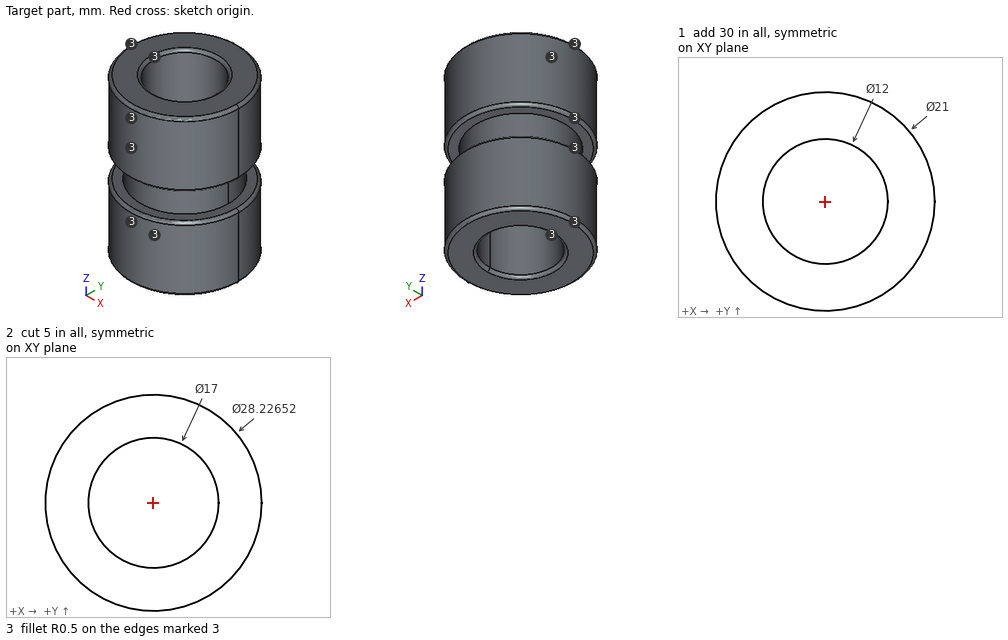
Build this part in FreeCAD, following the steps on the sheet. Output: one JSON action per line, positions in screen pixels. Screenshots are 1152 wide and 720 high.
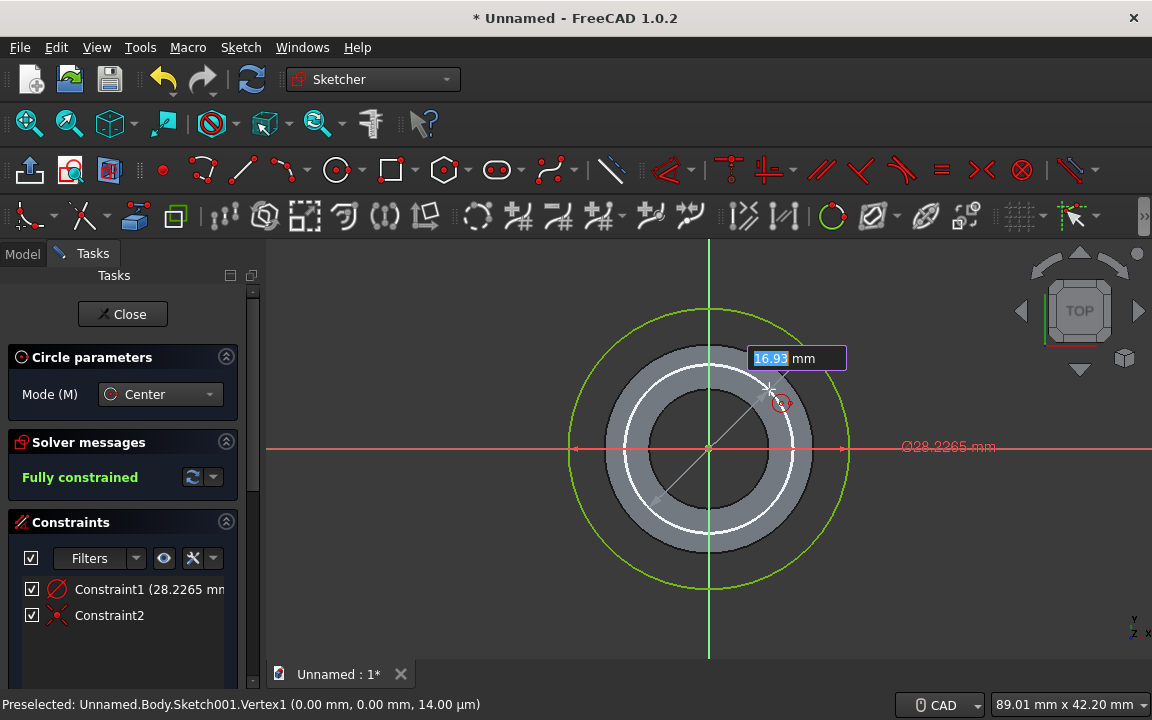
{"action": "type", "text": "17"}
{"action": "key", "text": "Return"}
{"action": "key", "text": "Escape"}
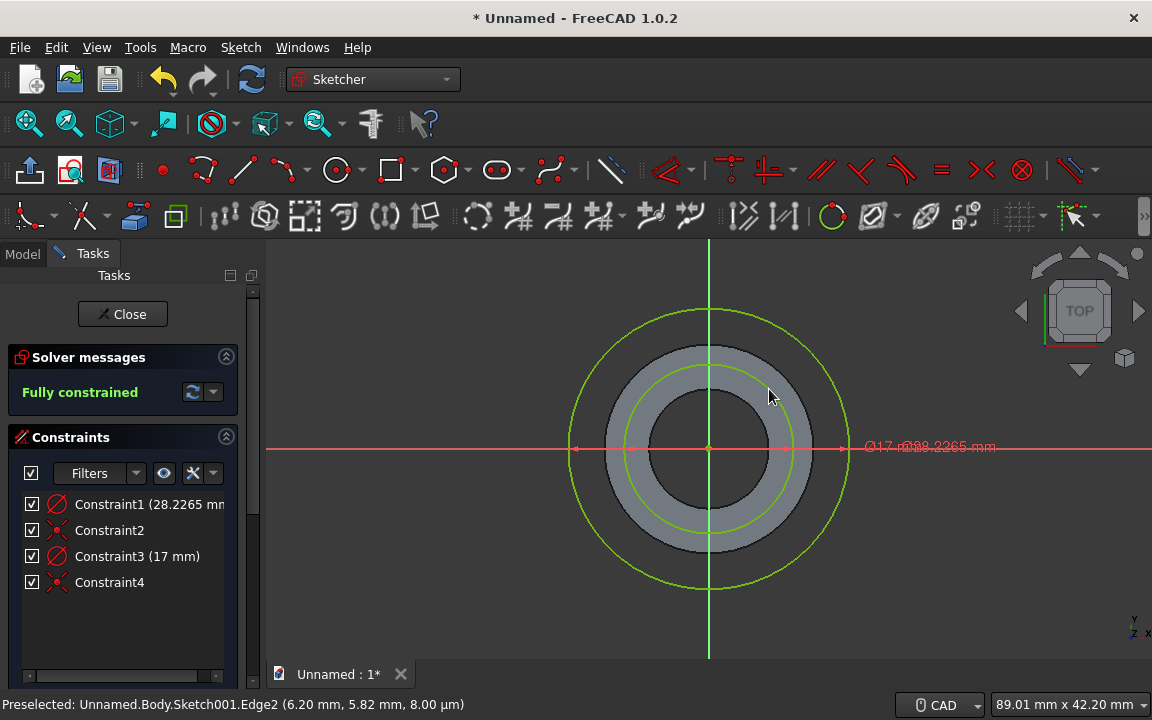
{"action": "left_click", "coordinate": [123, 314]}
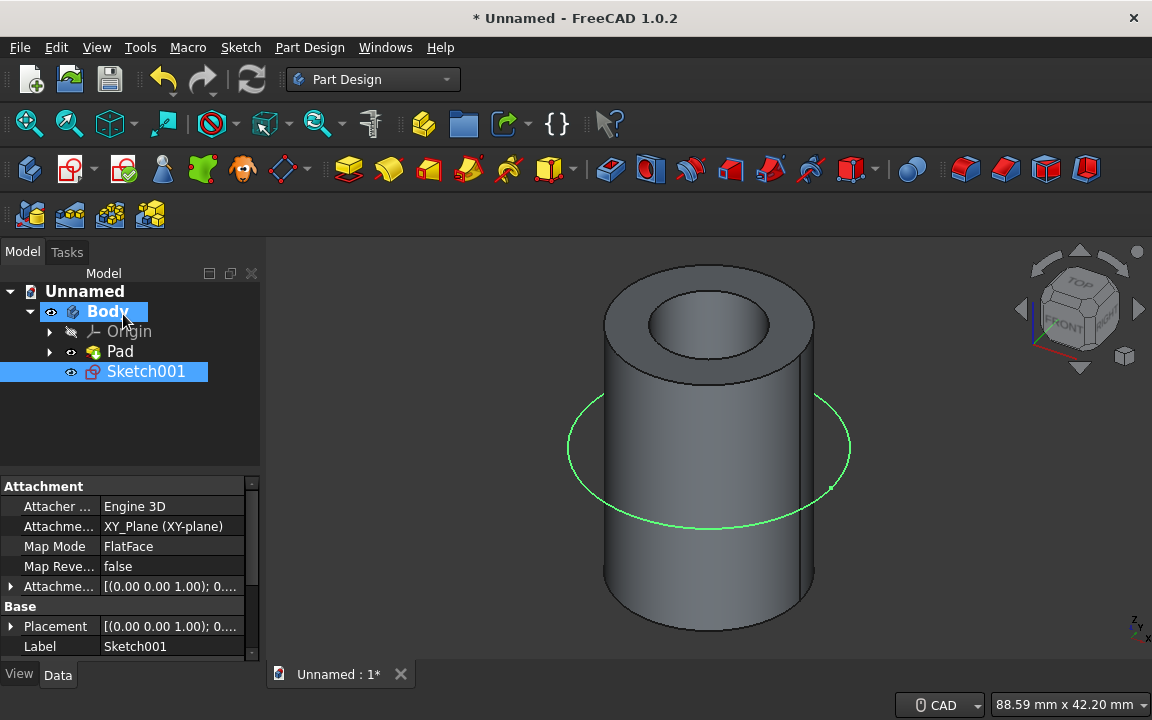
{"action": "left_click", "coordinate": [612, 170]}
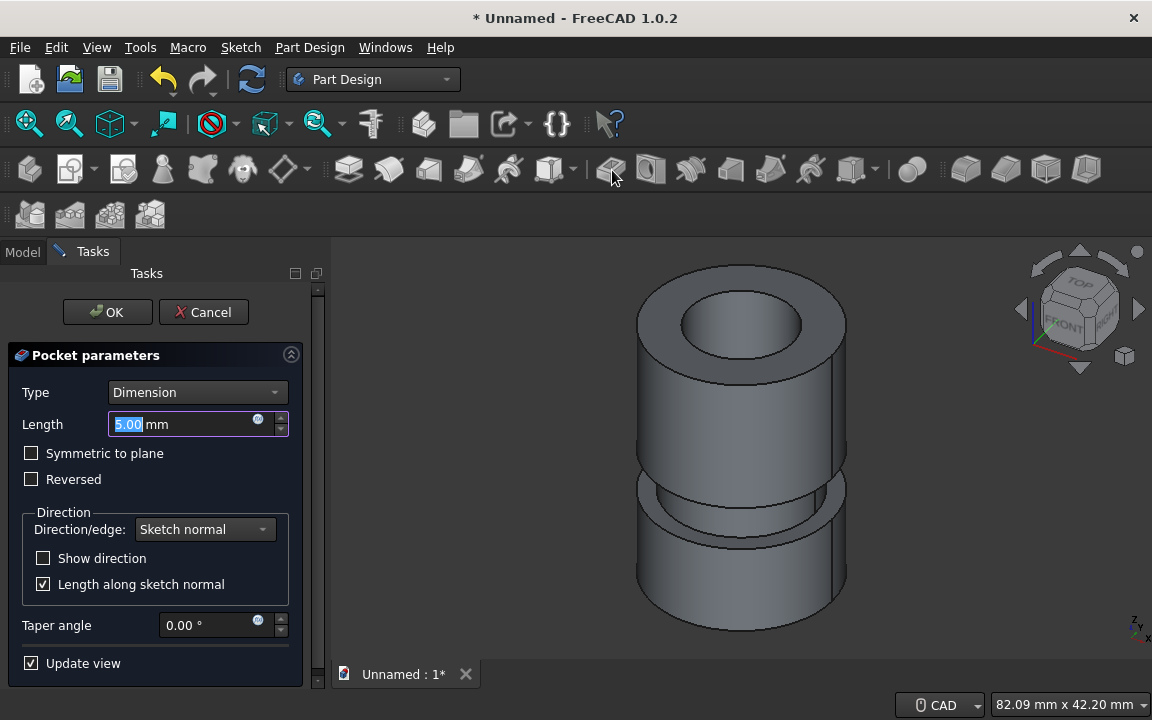
{"action": "type", "text": "5"}
{"action": "key", "text": "Tab"}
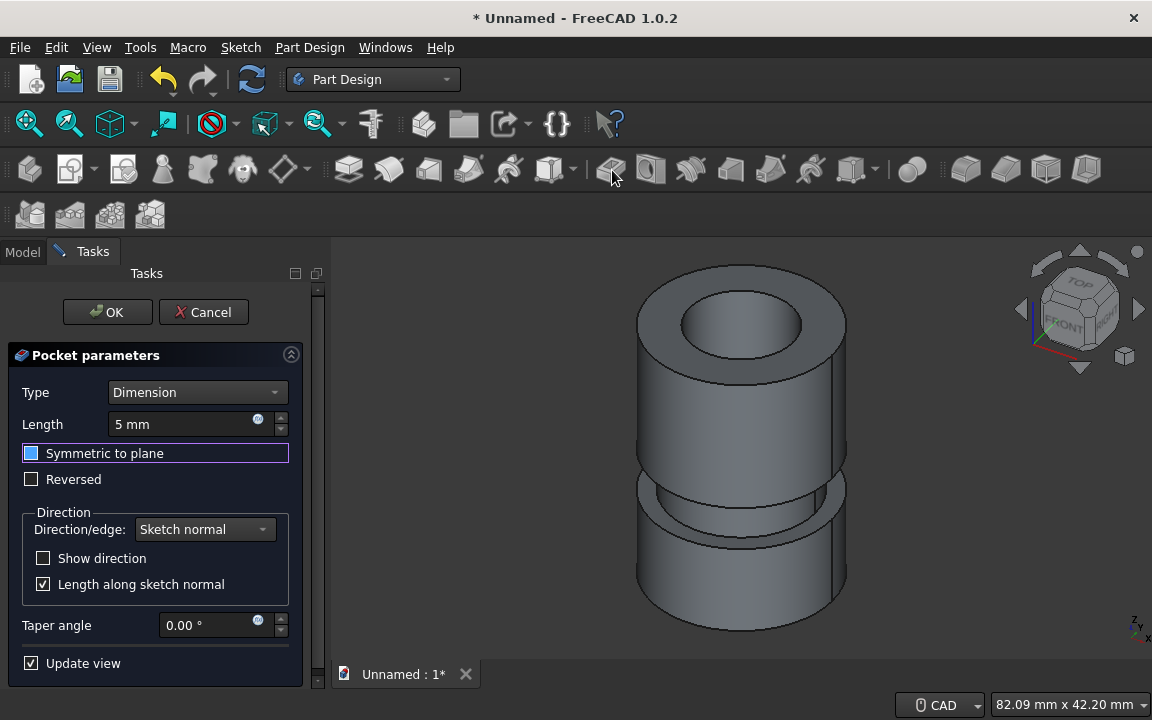
{"action": "left_click", "coordinate": [30, 453]}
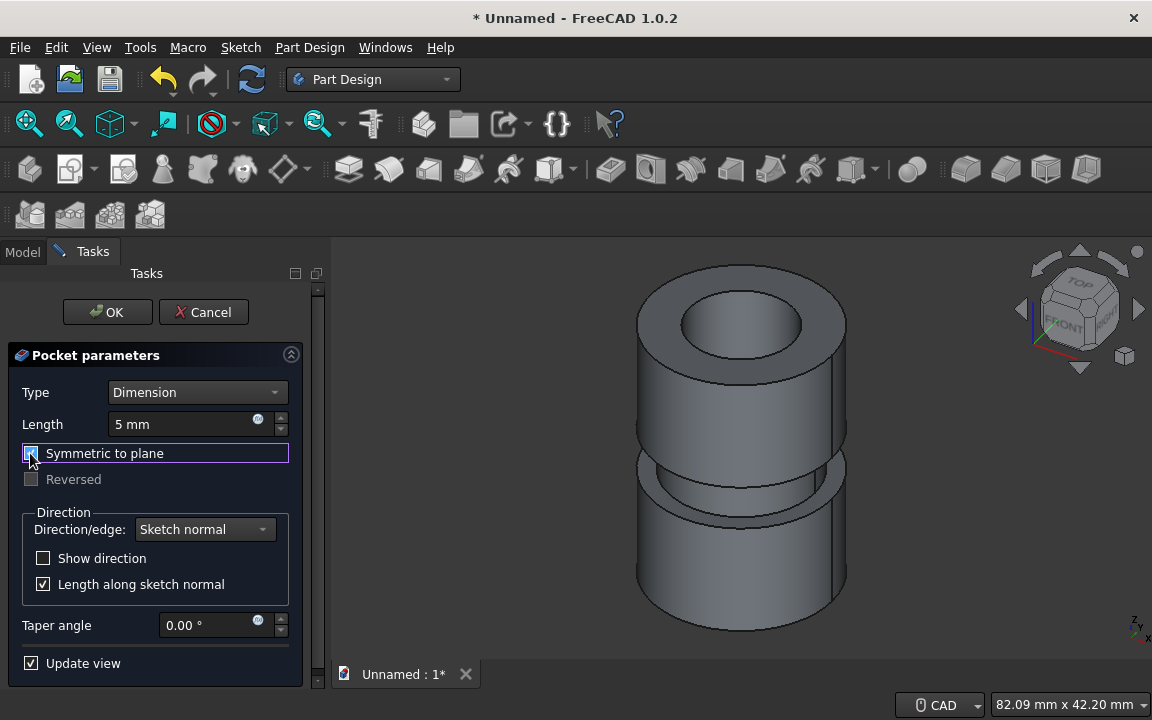
{"action": "left_click", "coordinate": [108, 312]}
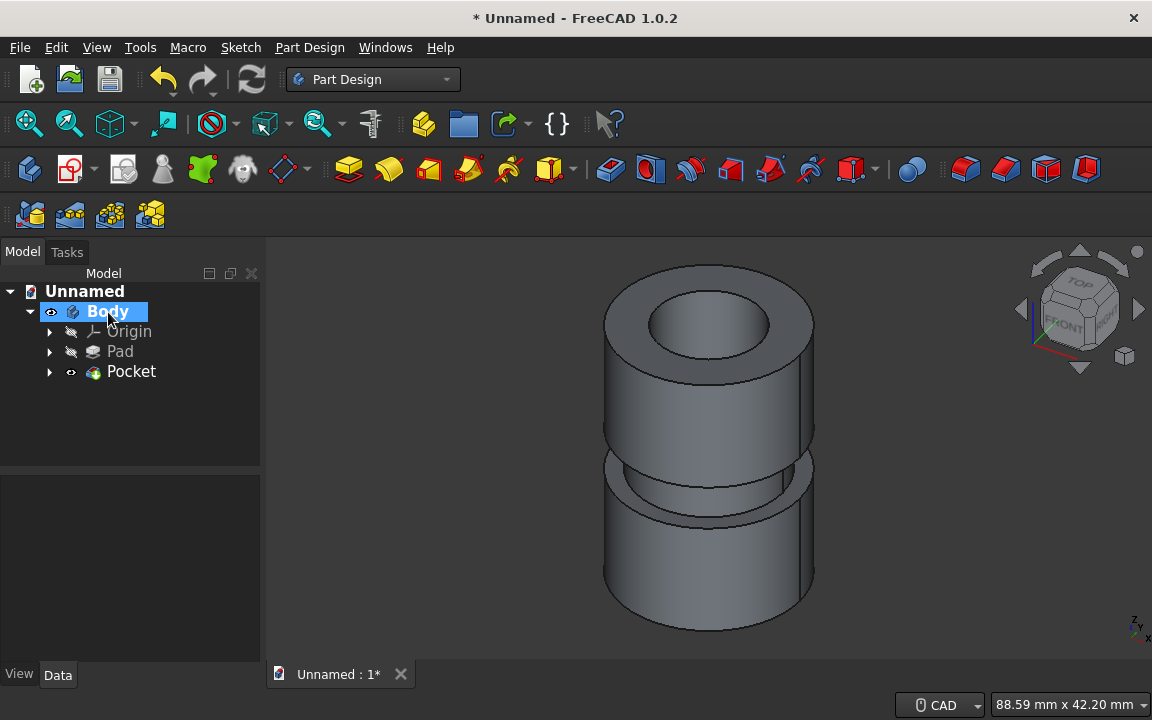
{"action": "left_click", "coordinate": [604, 474]}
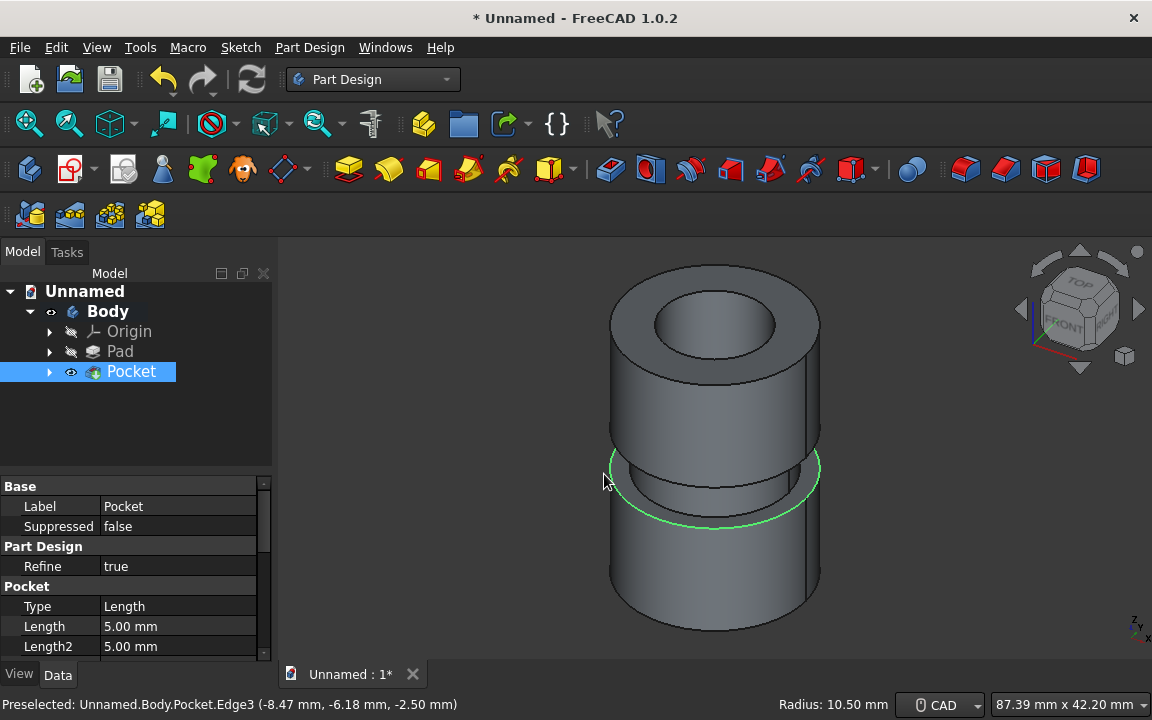
{"action": "left_click", "coordinate": [610, 330], "text": "ctrl"}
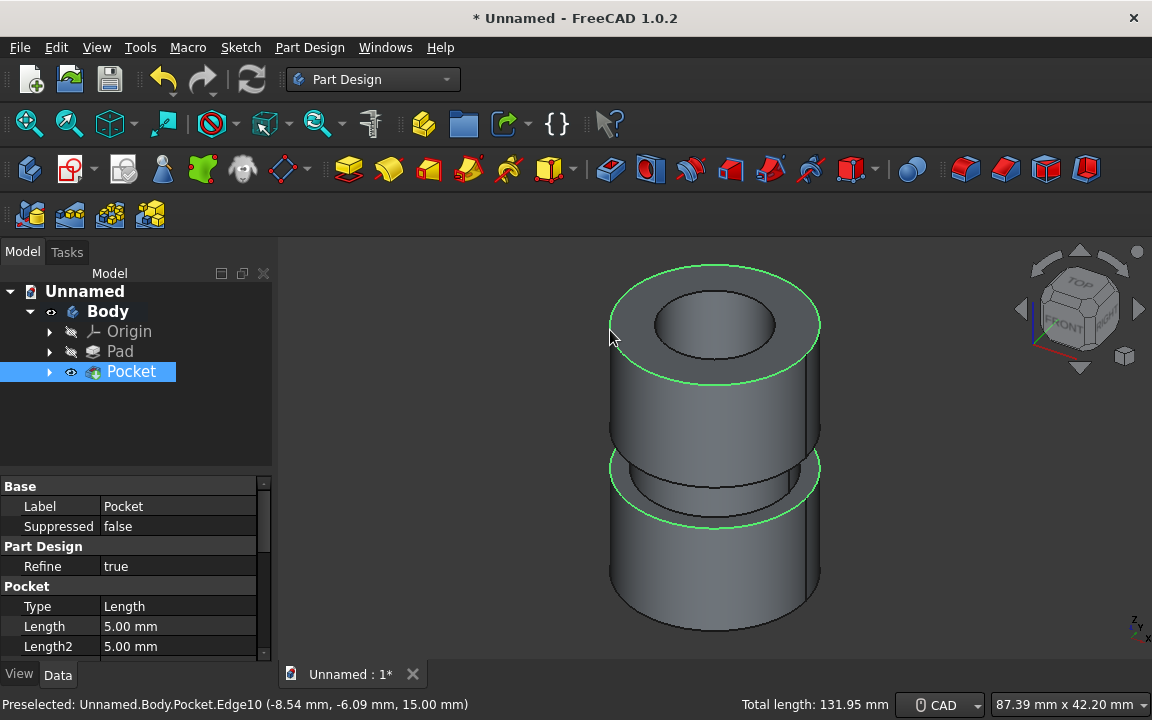
{"action": "left_click", "coordinate": [663, 307], "text": "ctrl"}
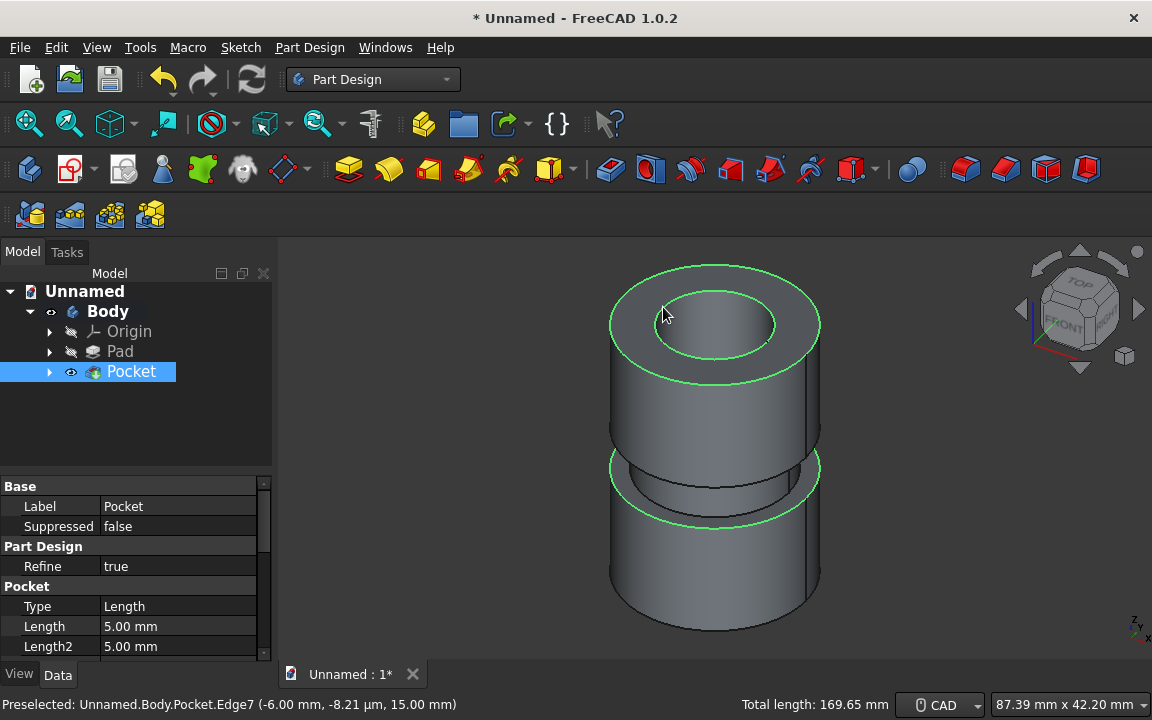
{"action": "key", "text": "0"}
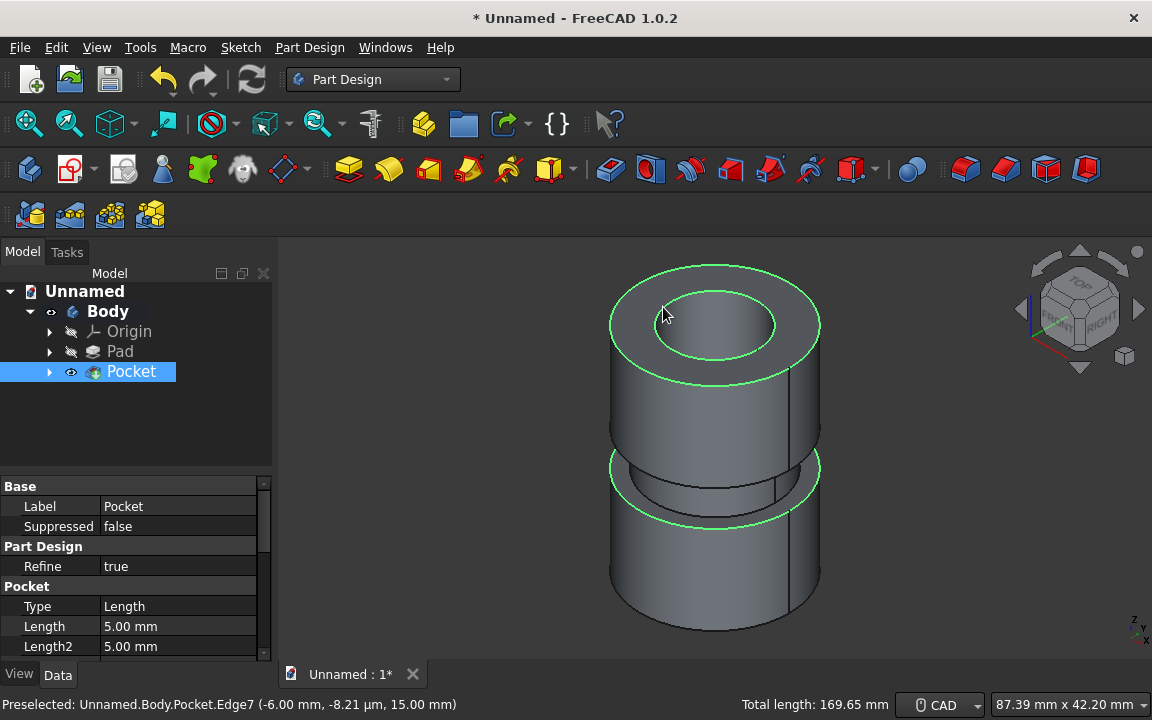
{"action": "key", "text": "2"}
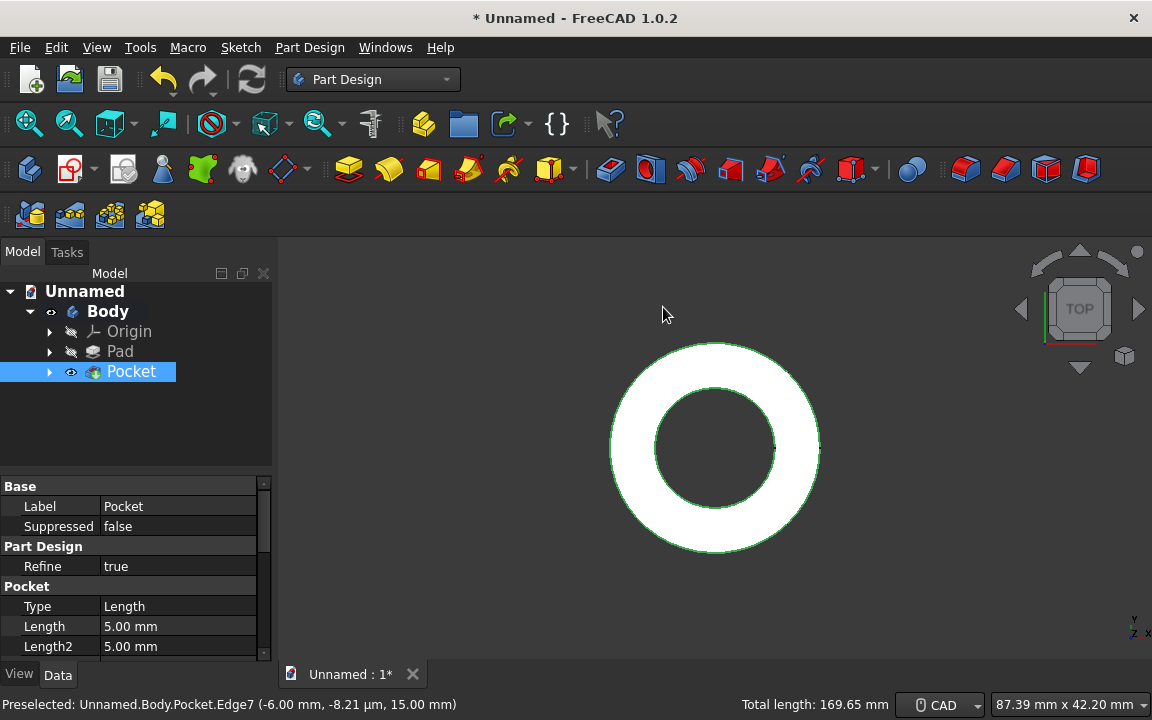
{"action": "key", "text": "1"}